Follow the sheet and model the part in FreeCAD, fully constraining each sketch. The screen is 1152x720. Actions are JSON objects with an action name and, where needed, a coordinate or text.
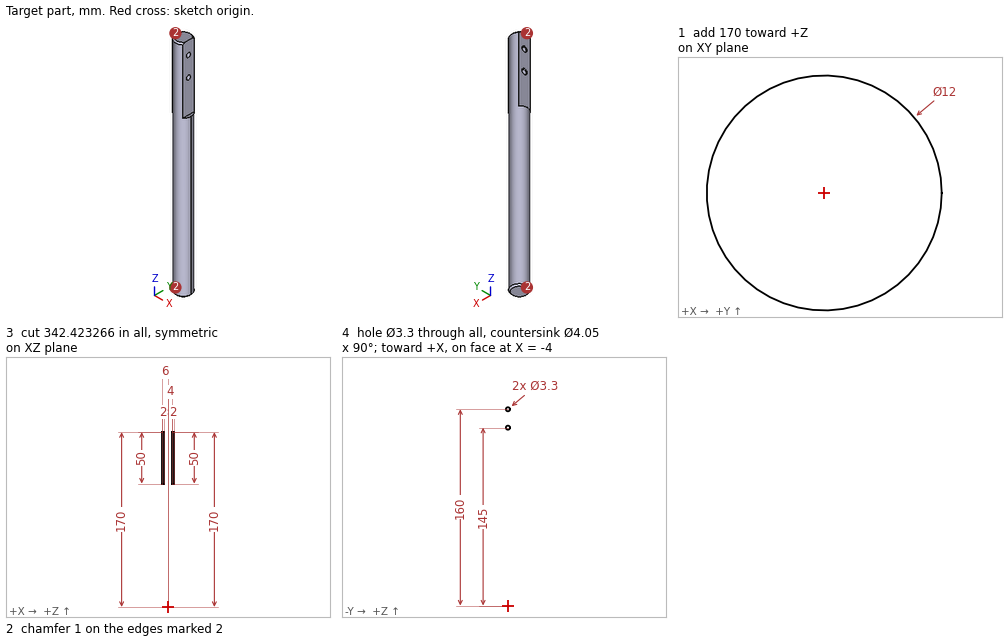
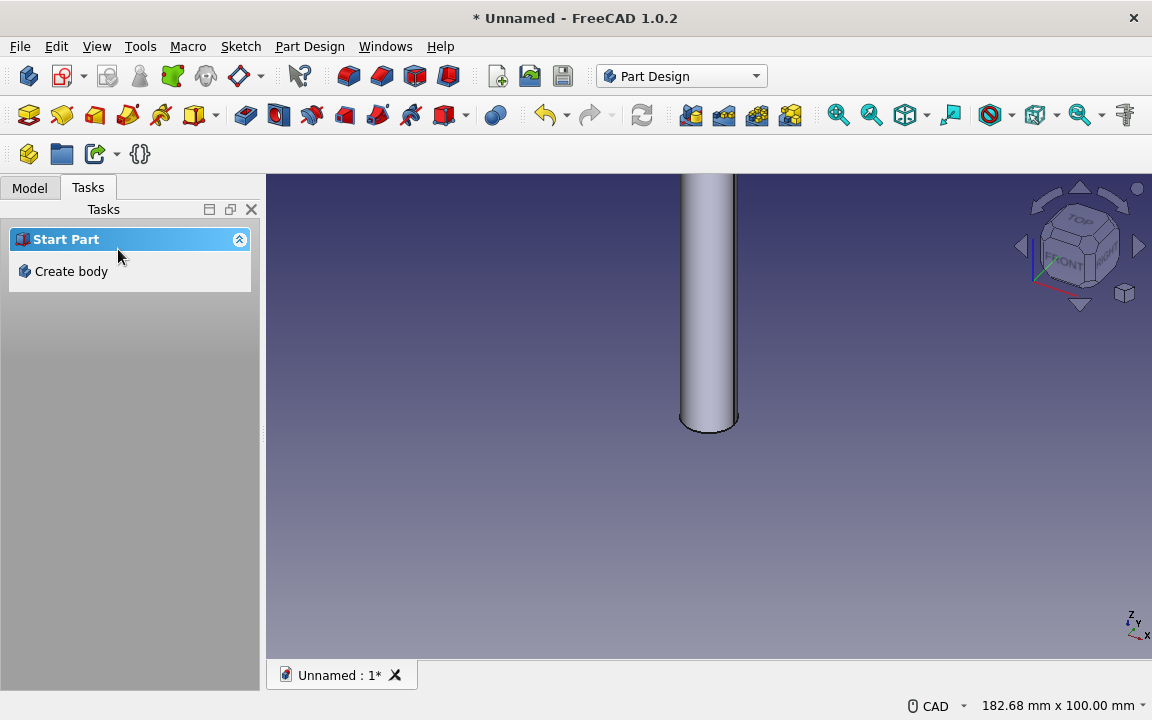
{"action": "key", "text": "v f"}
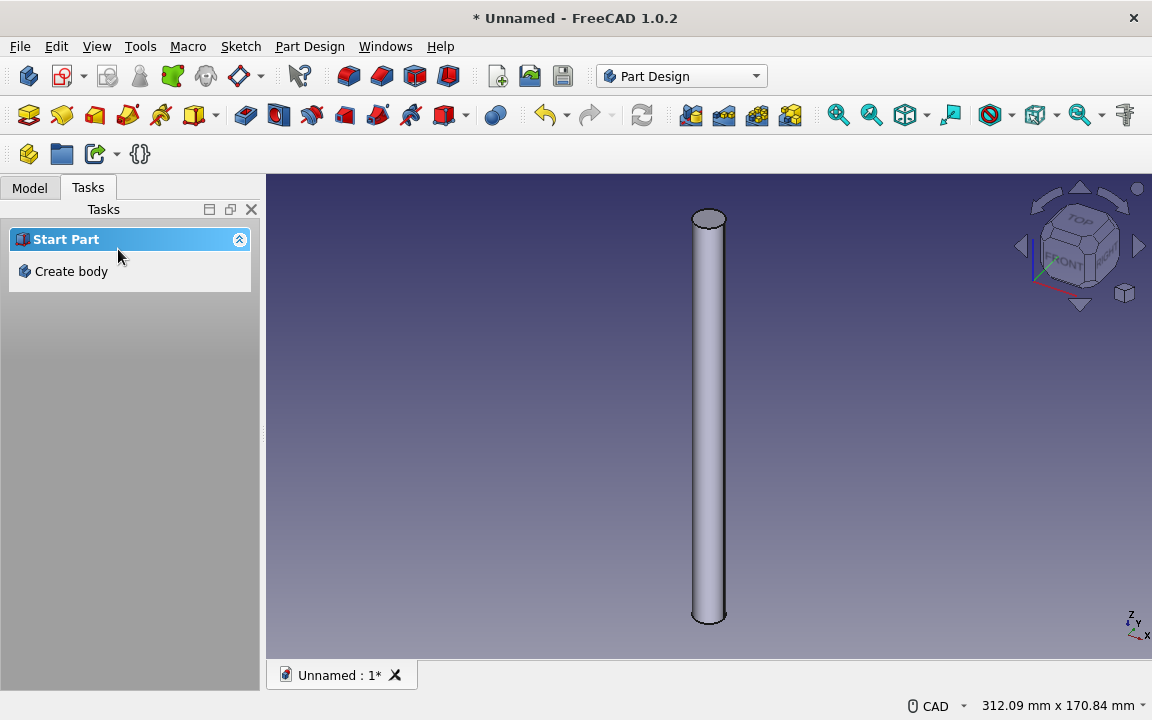
{"action": "left_click", "coordinate": [696, 620]}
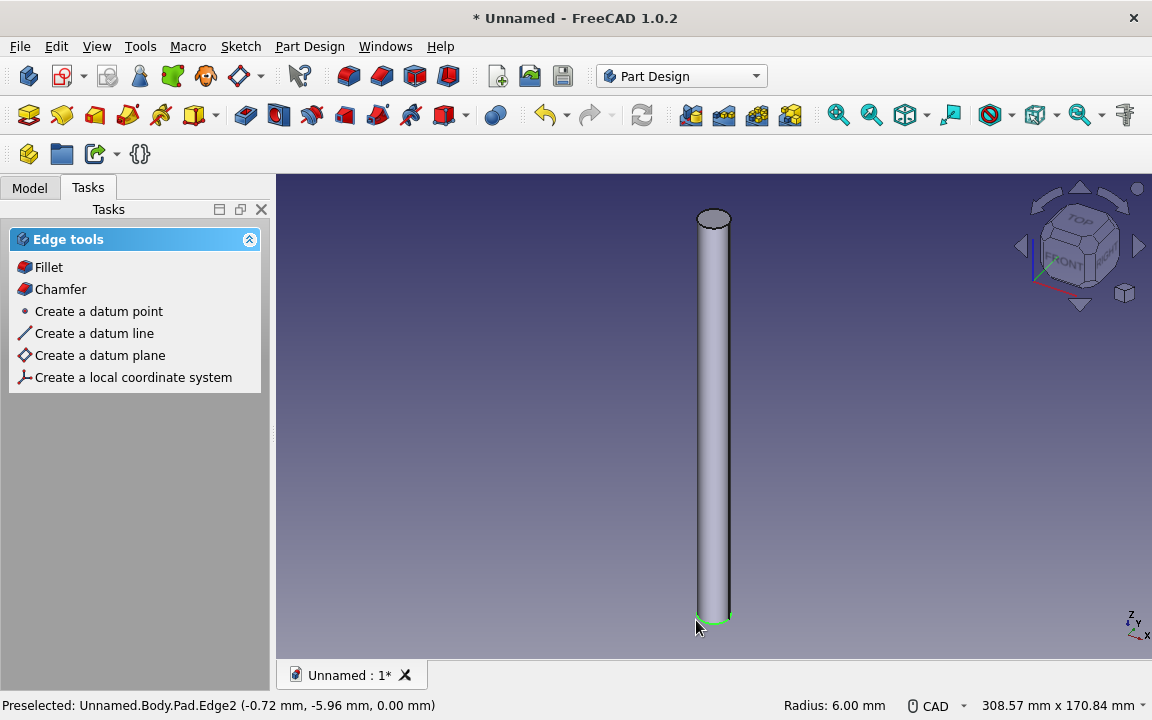
{"action": "left_click", "coordinate": [699, 213], "text": "ctrl"}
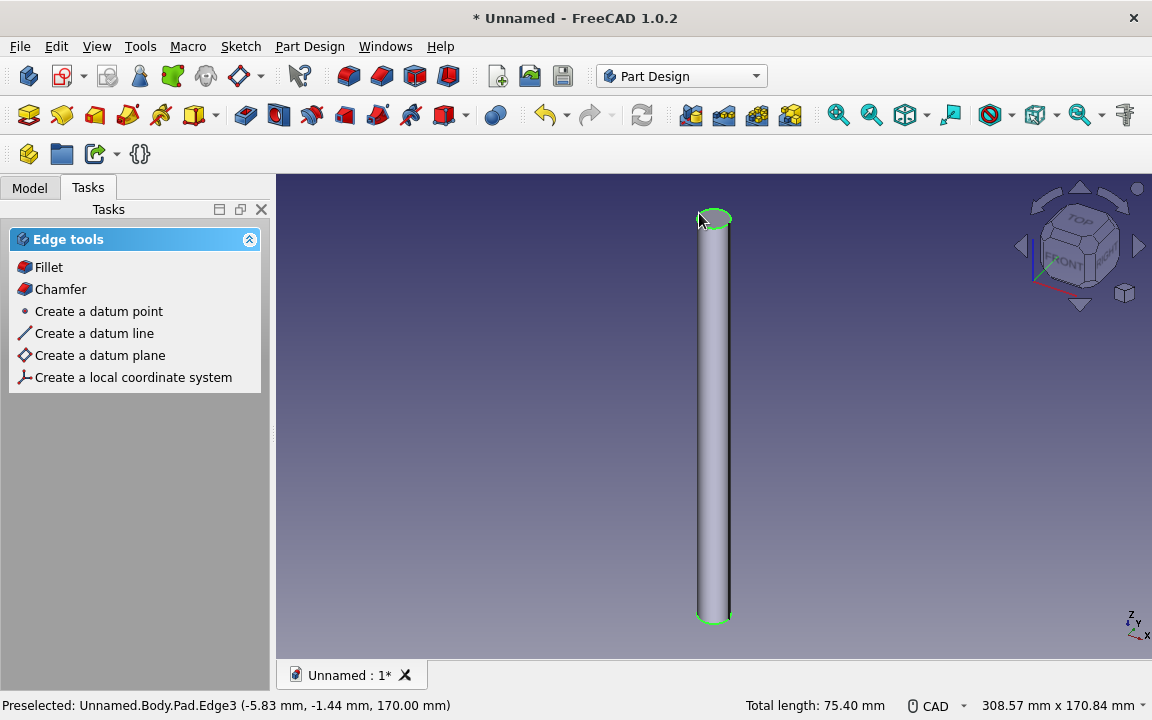
{"action": "left_click", "coordinate": [382, 76]}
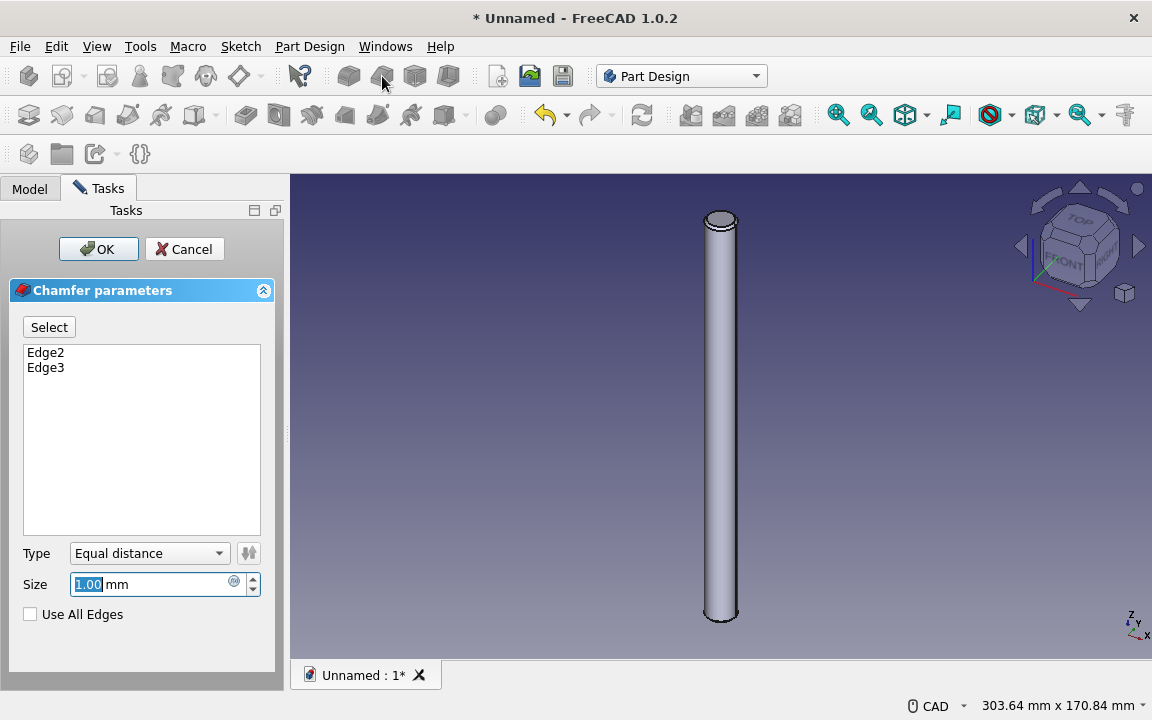
{"action": "type", "text": "1"}
{"action": "key", "text": "Tab"}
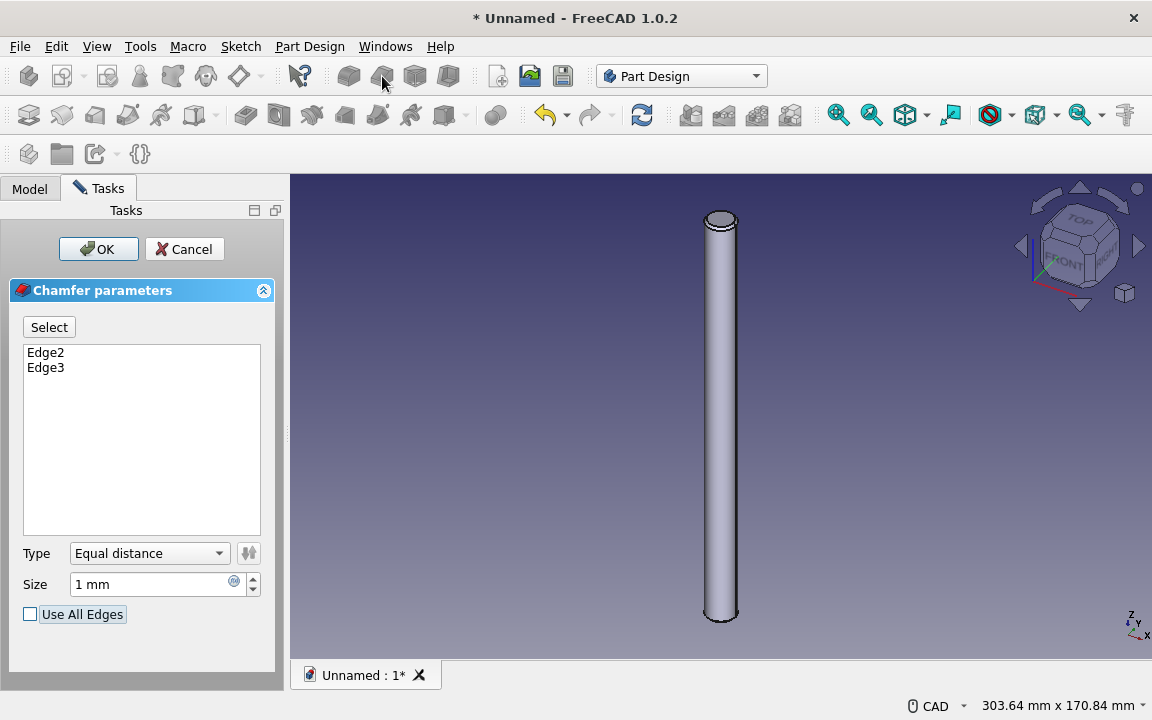
{"action": "left_click", "coordinate": [99, 249]}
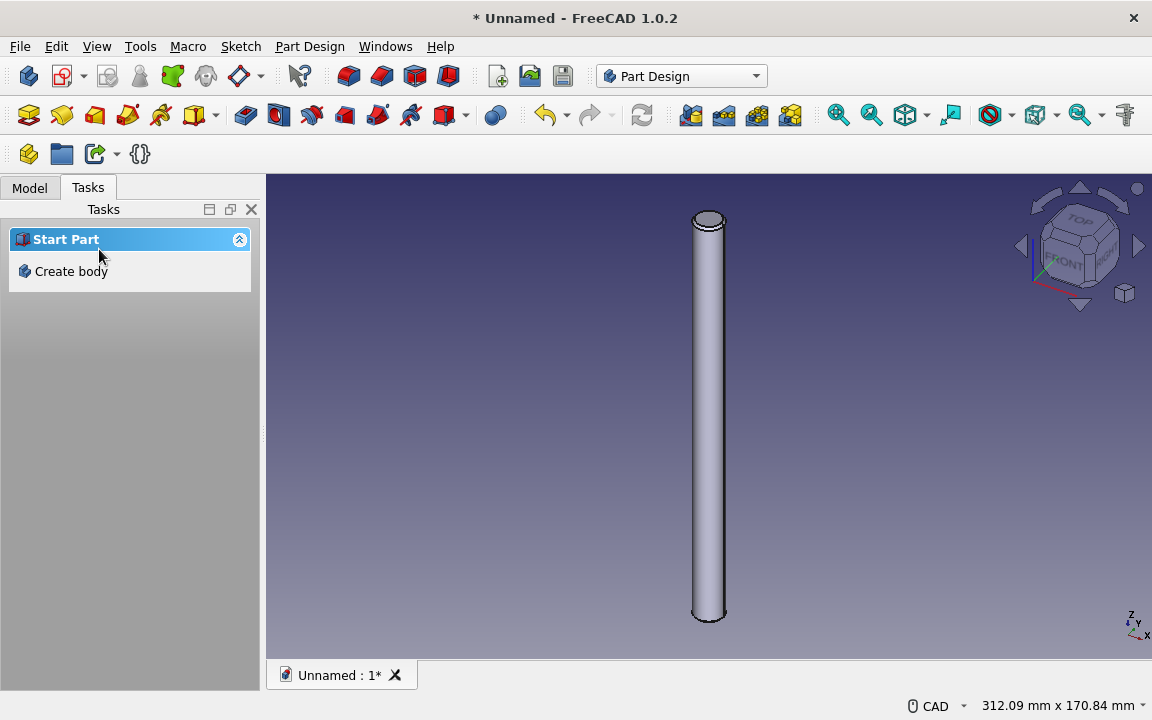
{"action": "left_click", "coordinate": [62, 76]}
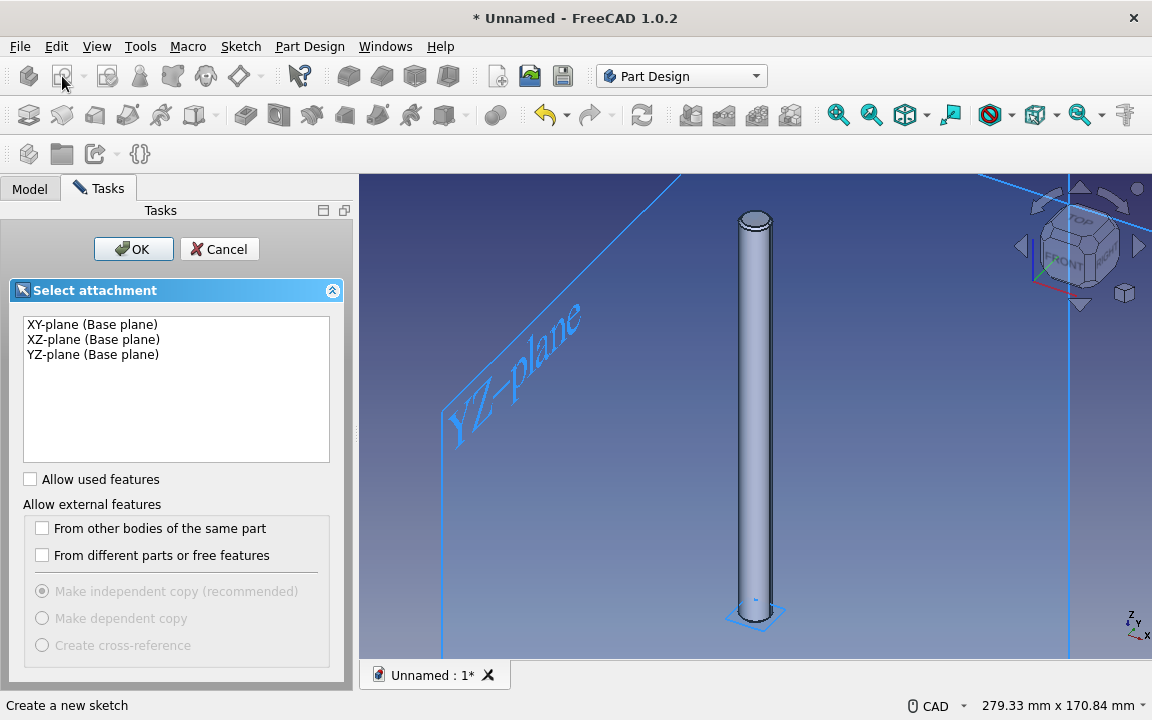
{"action": "left_click", "coordinate": [84, 340]}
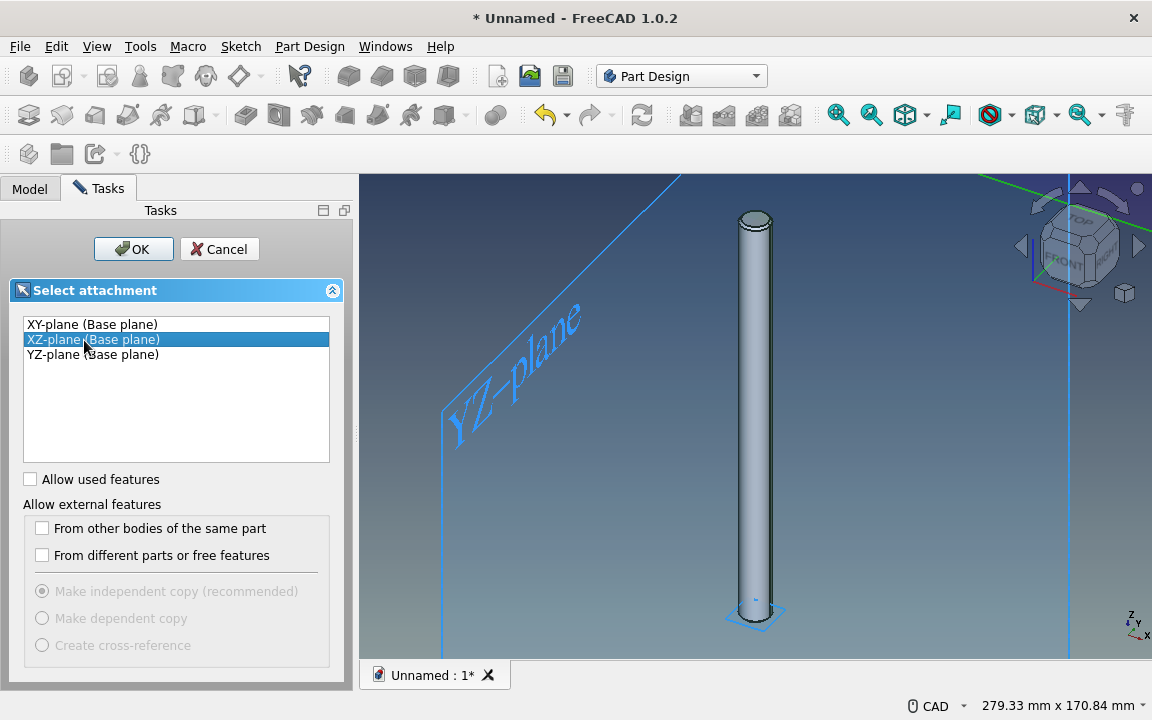
{"action": "left_click", "coordinate": [134, 249]}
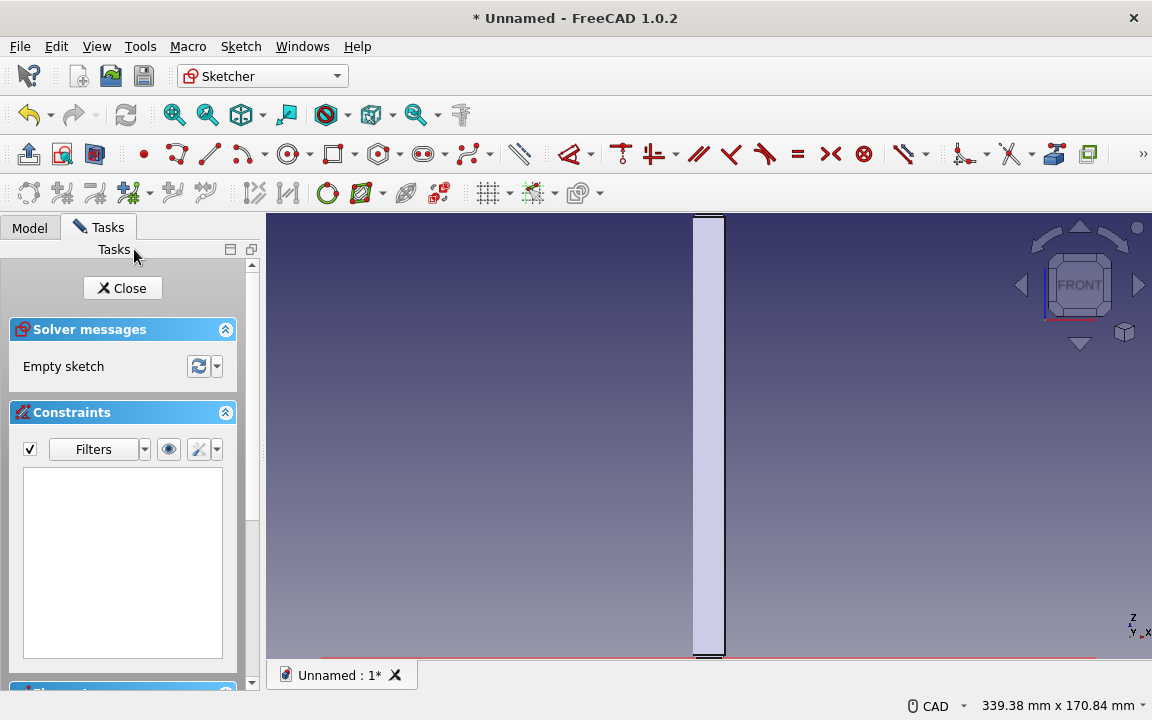
{"action": "left_click", "coordinate": [95, 154]}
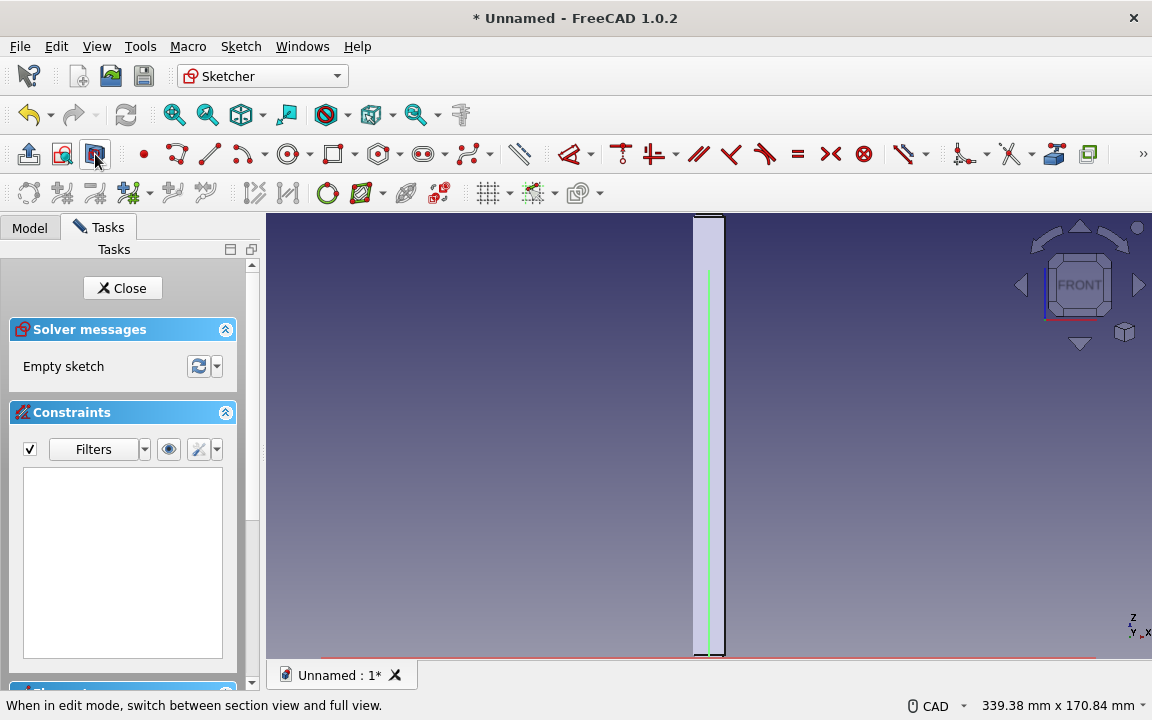
{"action": "scroll", "coordinate": [640, 436], "scroll_direction": "down", "scroll_amount": 5}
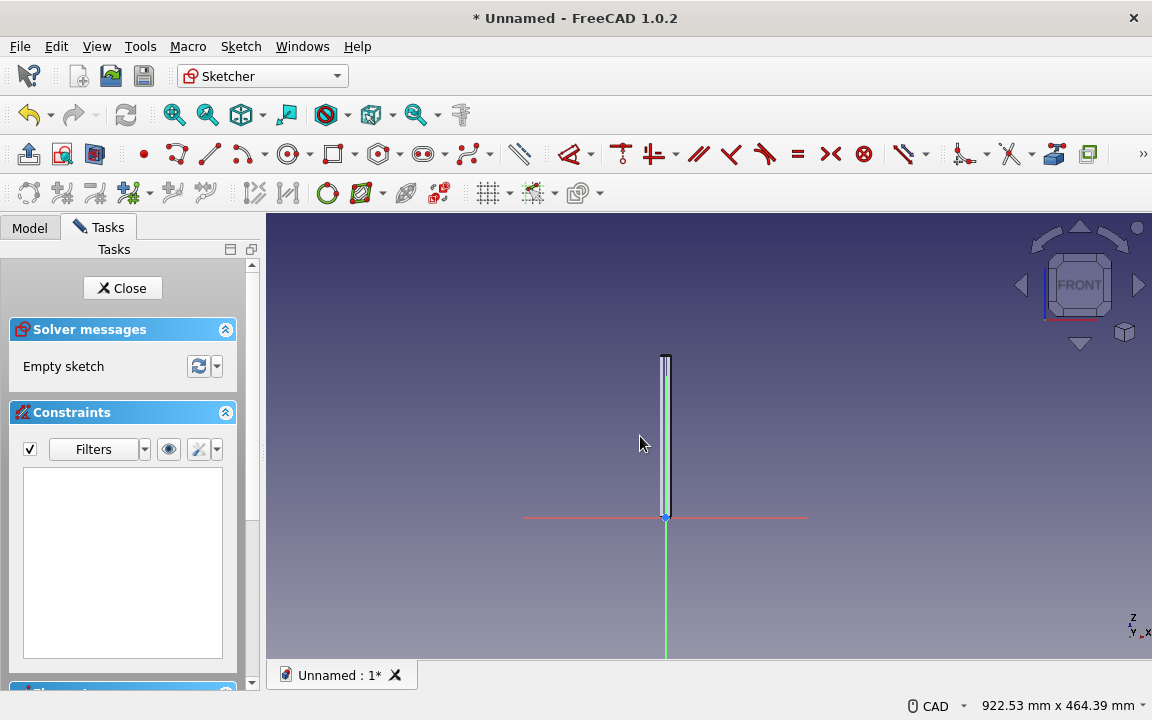
{"action": "scroll", "coordinate": [671, 367], "scroll_direction": "up", "scroll_amount": 9}